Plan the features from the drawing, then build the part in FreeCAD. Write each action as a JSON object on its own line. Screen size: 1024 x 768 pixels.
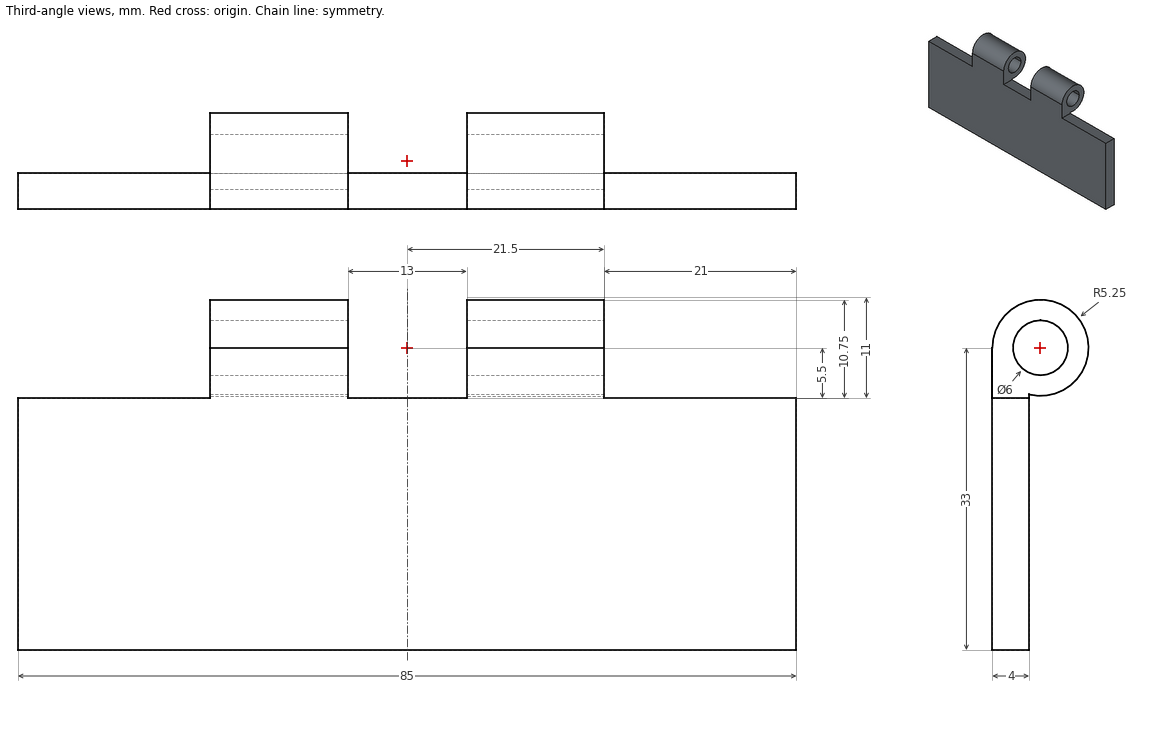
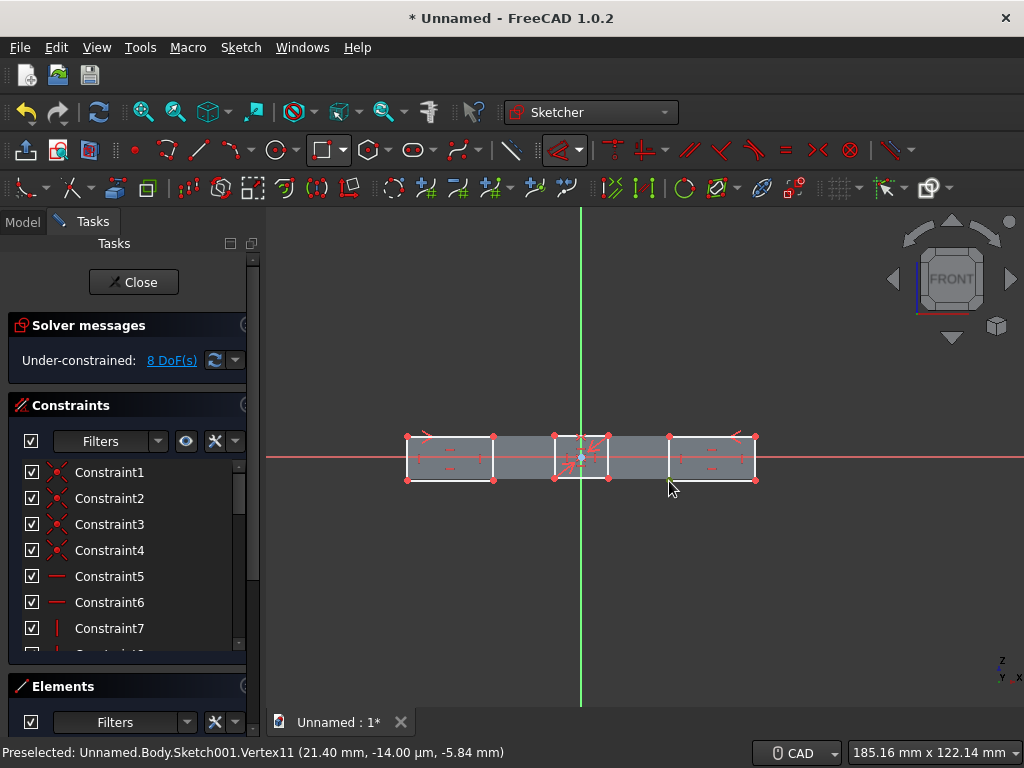
{"action": "left_click", "coordinate": [493, 481]}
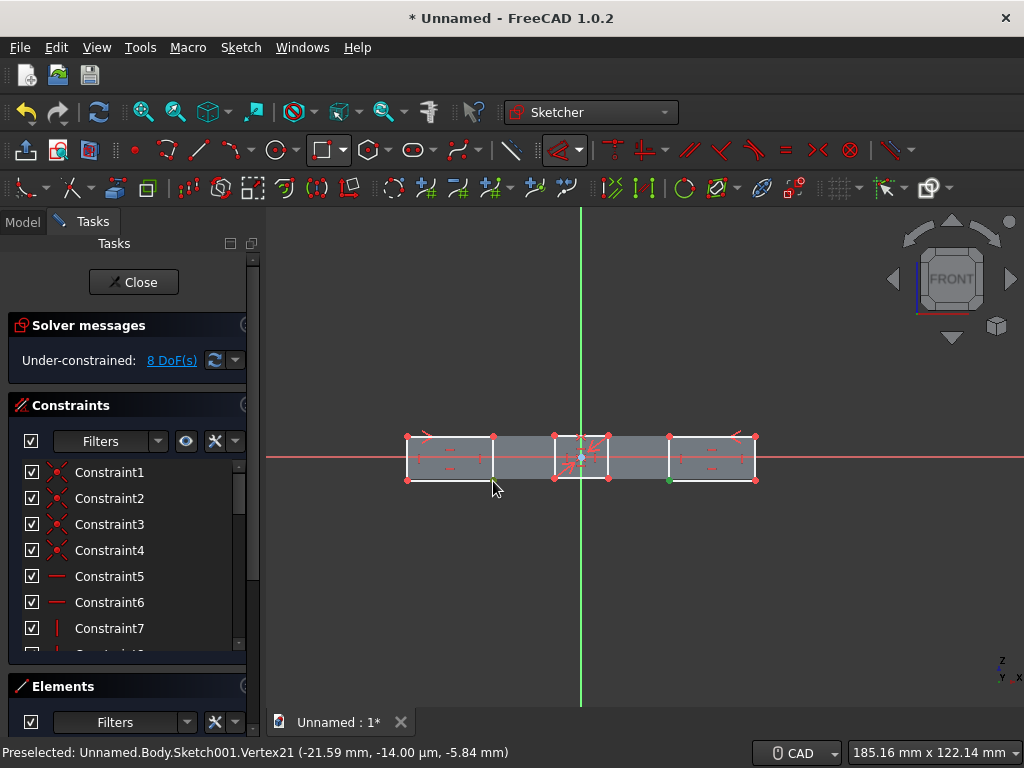
{"action": "left_click", "coordinate": [581, 647]}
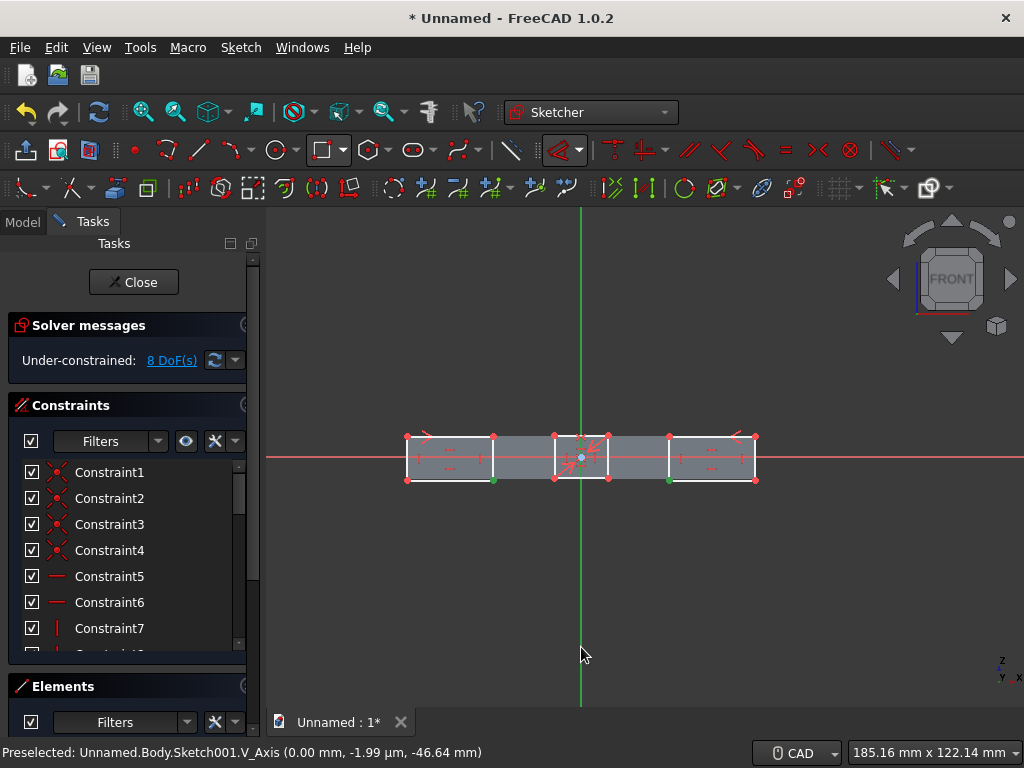
{"action": "left_click", "coordinate": [818, 150]}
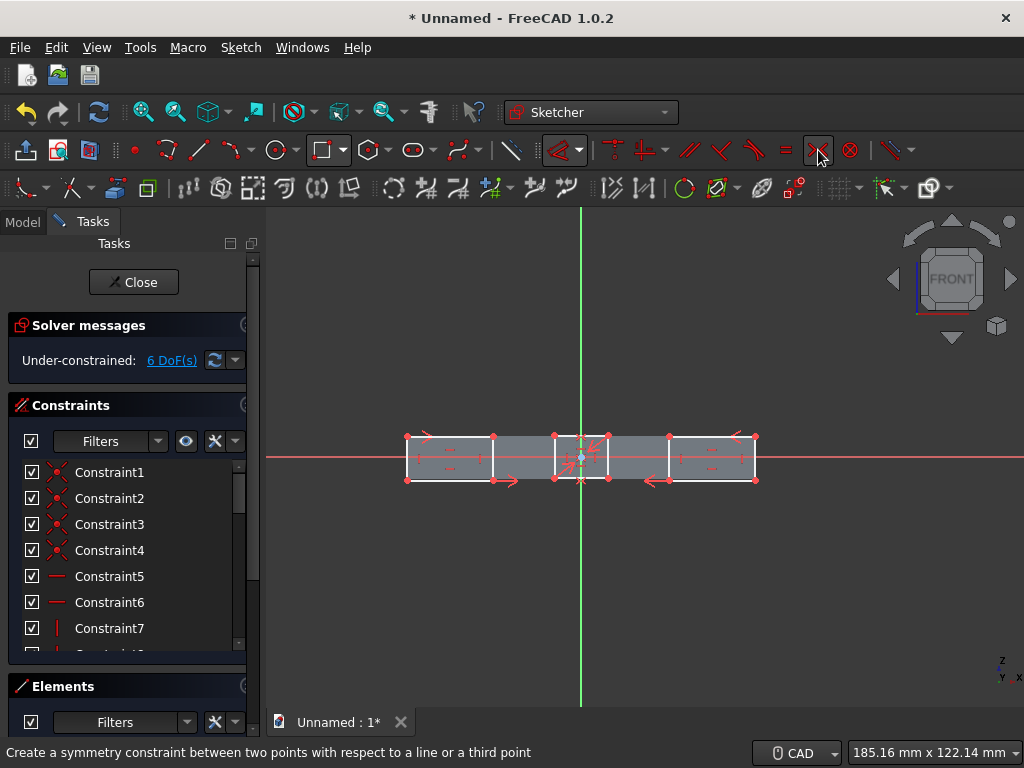
{"action": "scroll", "coordinate": [571, 478], "scroll_direction": "up", "scroll_amount": 2}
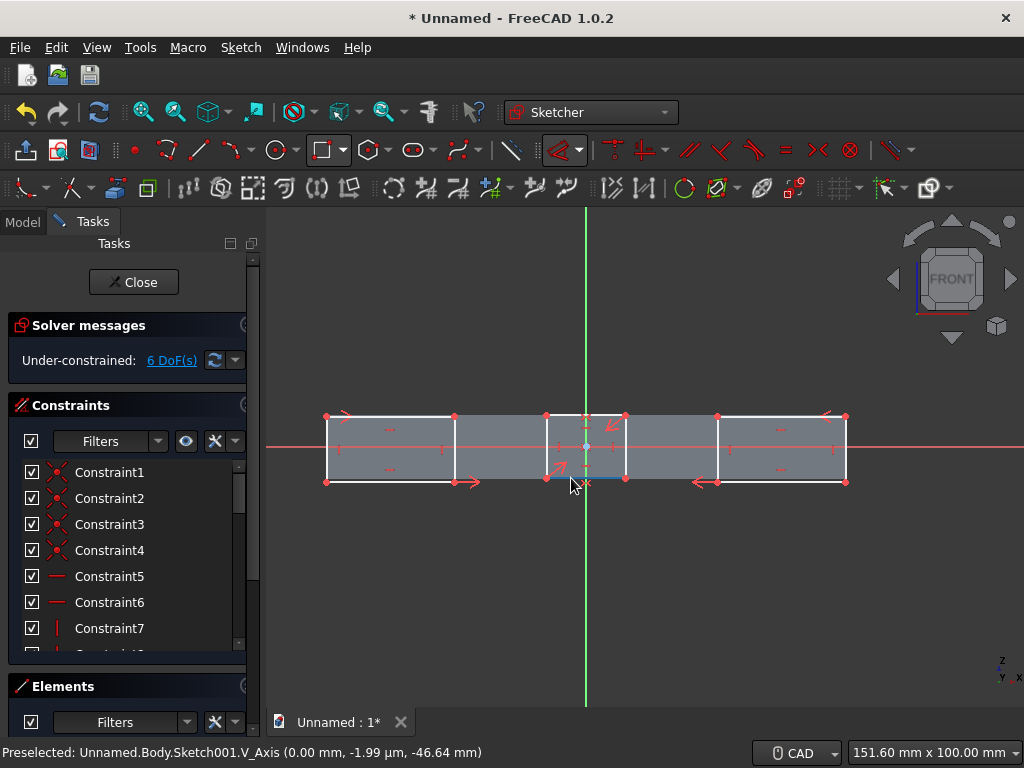
{"action": "left_click", "coordinate": [570, 478]}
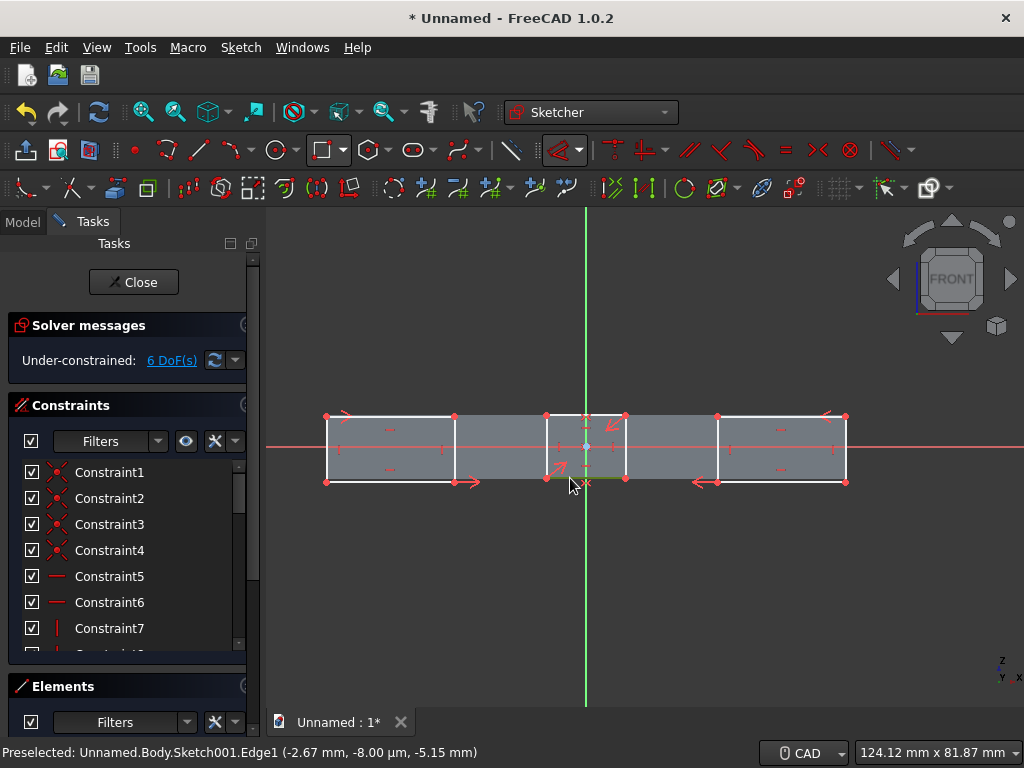
{"action": "key", "text": "l"}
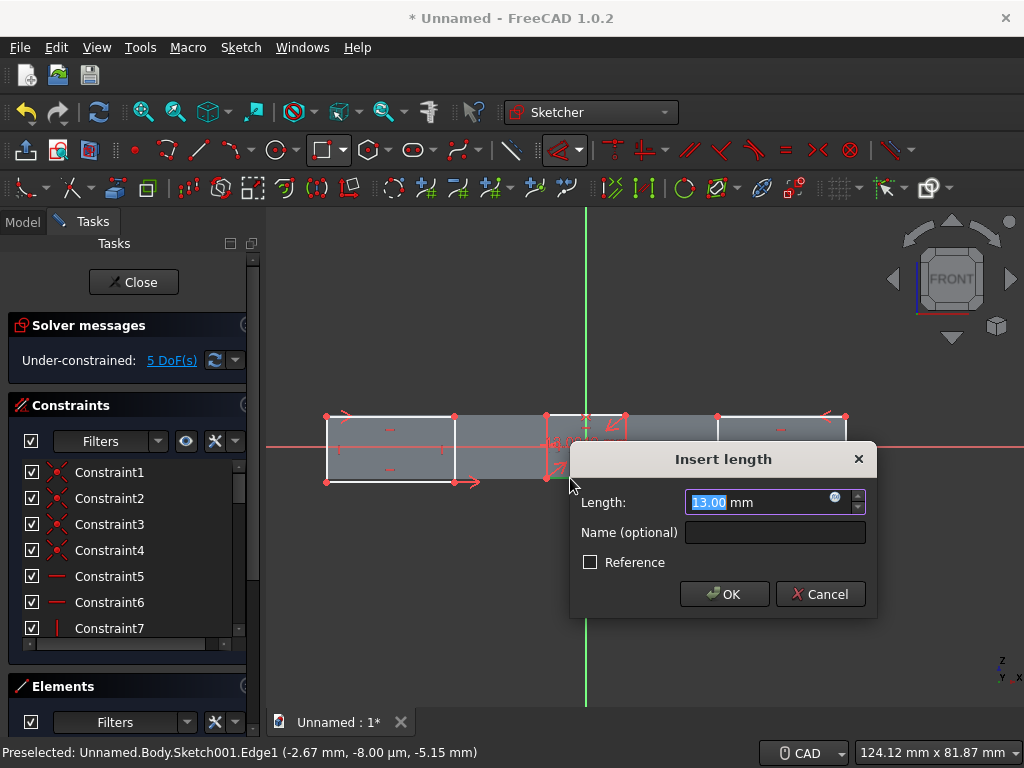
{"action": "type", "text": "13"}
{"action": "key", "text": "Return"}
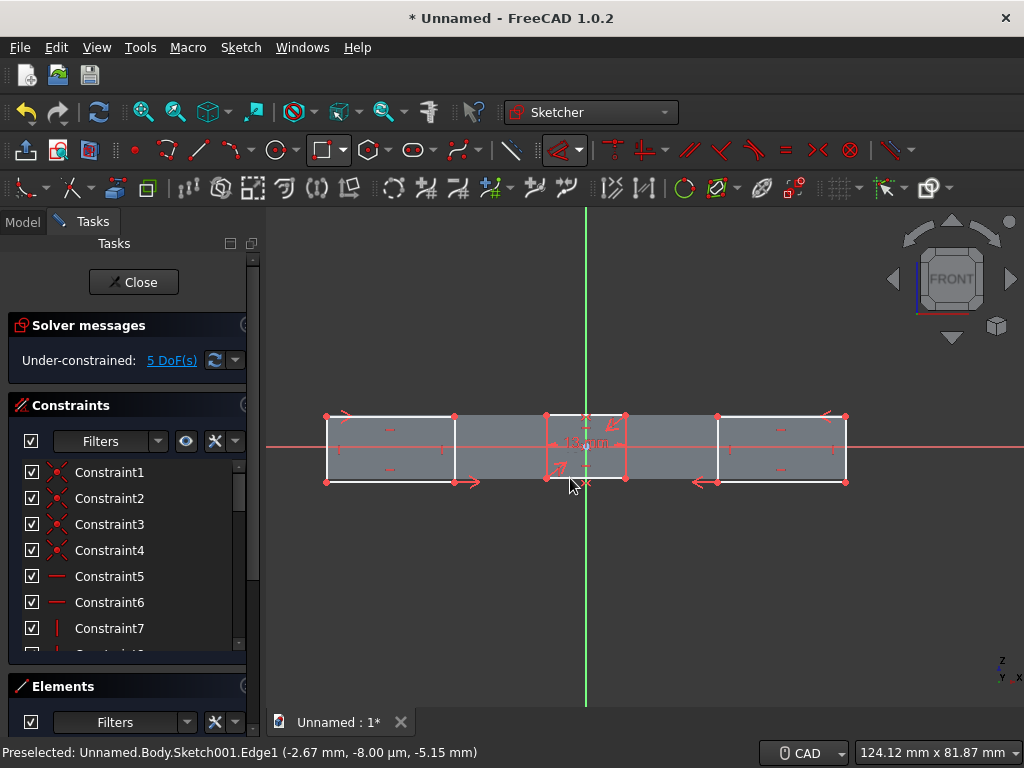
{"action": "left_click", "coordinate": [626, 459]}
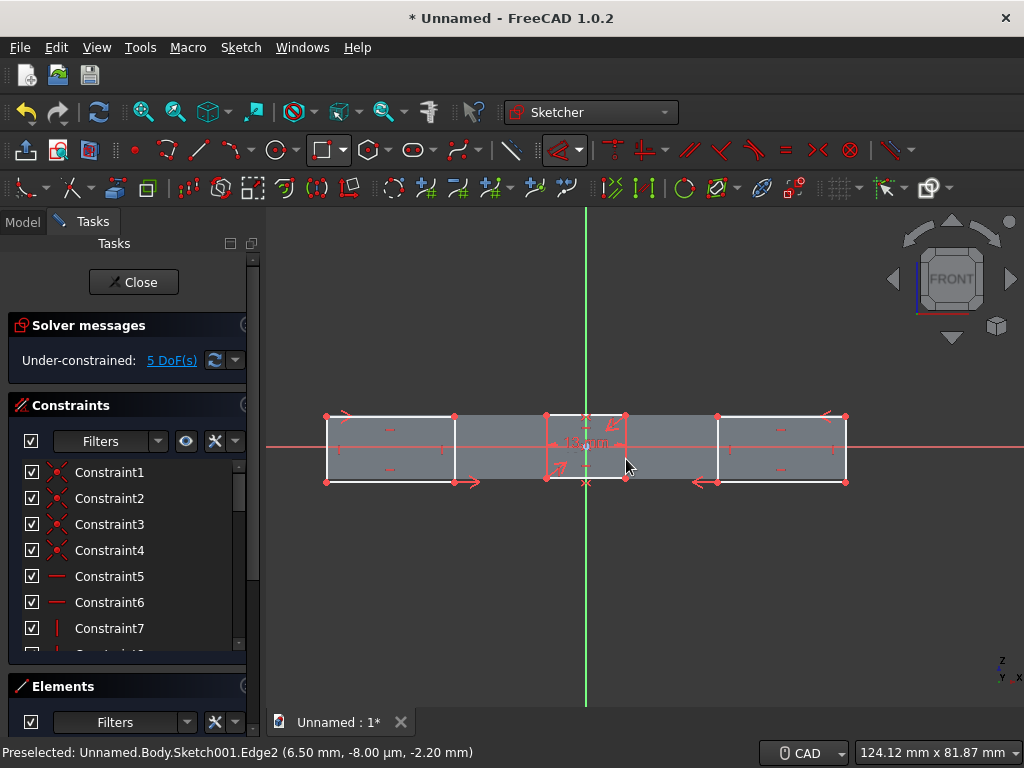
{"action": "left_click", "coordinate": [582, 150]}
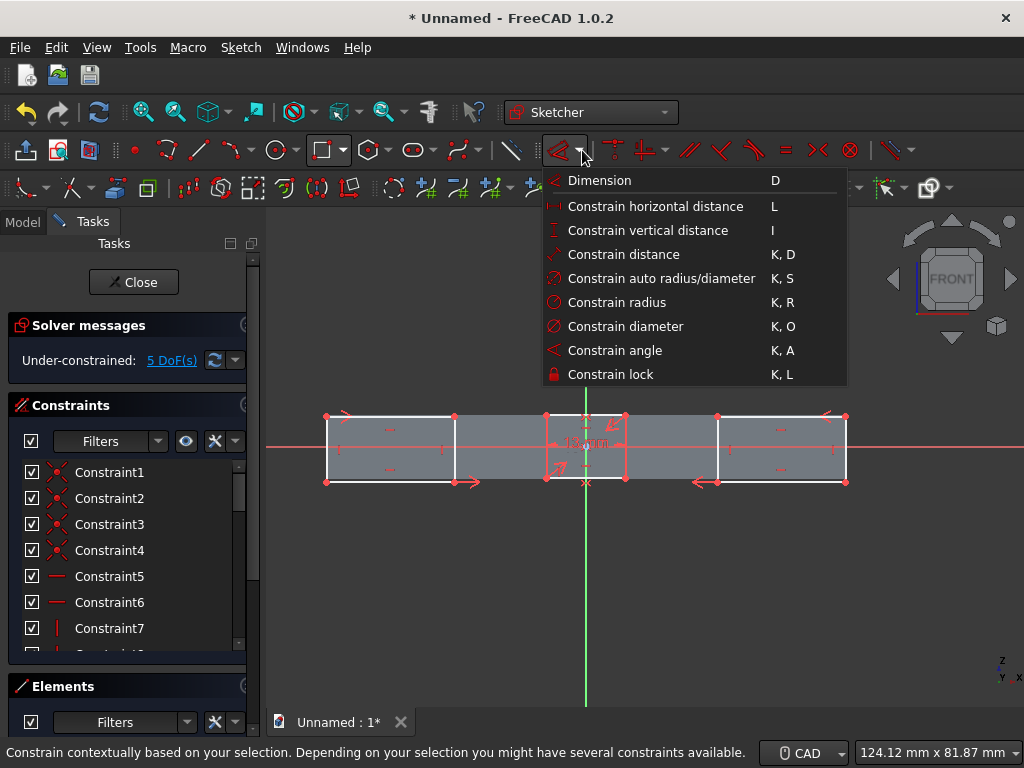
{"action": "left_click", "coordinate": [695, 230]}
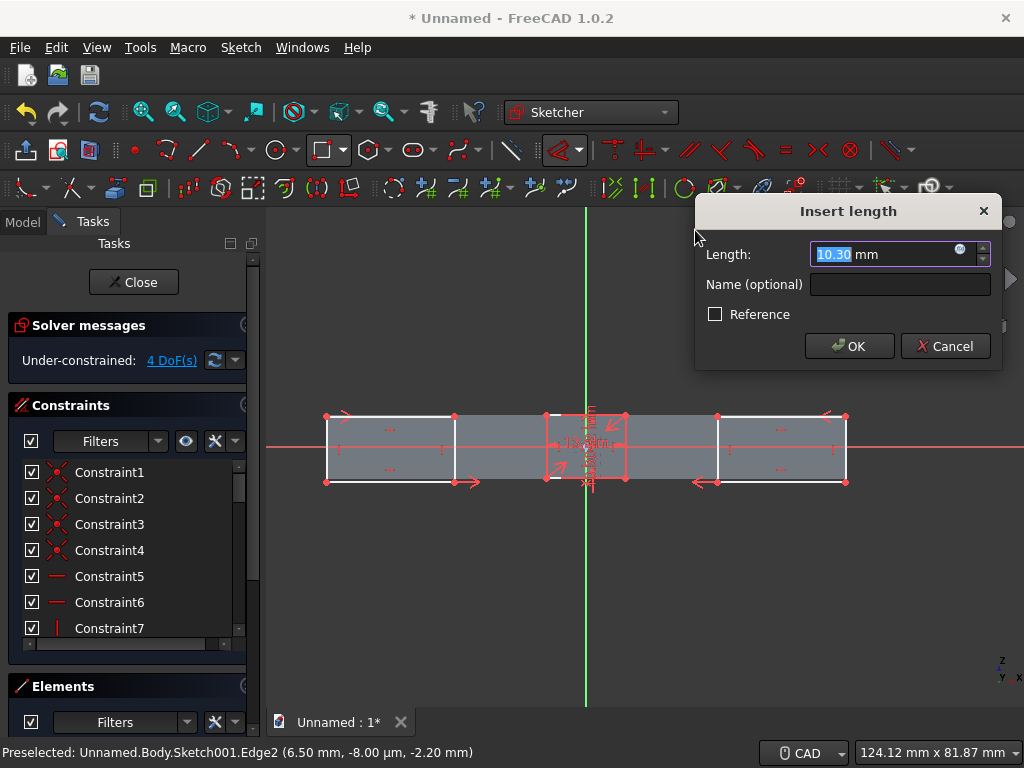
{"action": "type", "text": "11"}
{"action": "key", "text": "Return"}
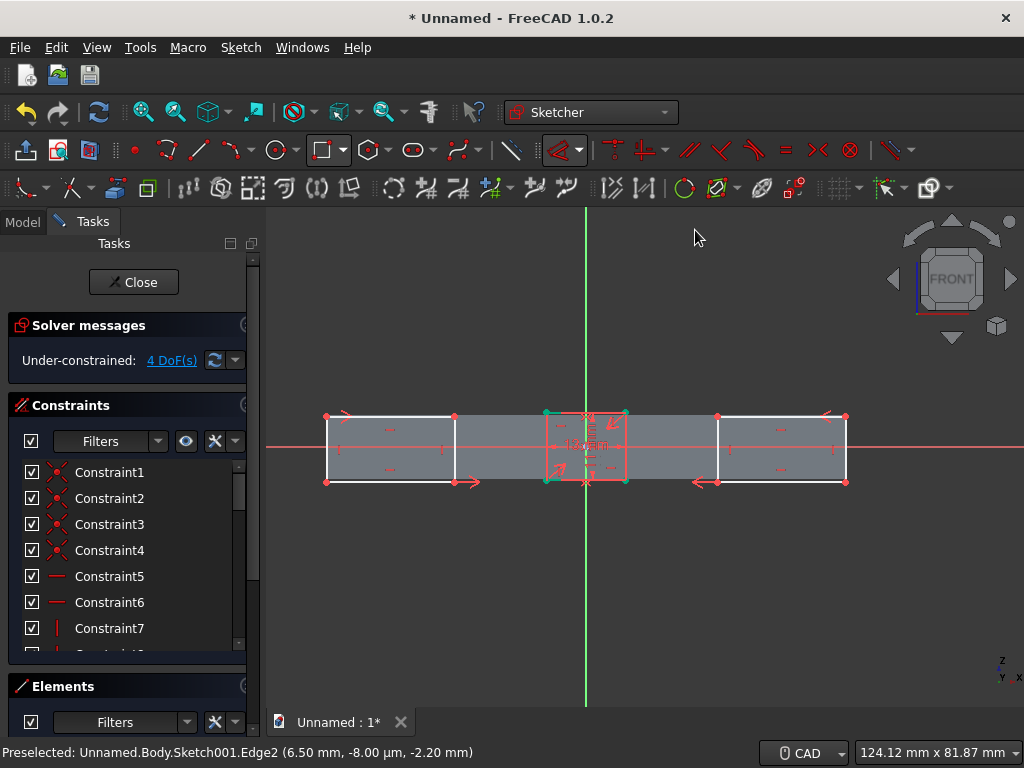
{"action": "left_click", "coordinate": [756, 482]}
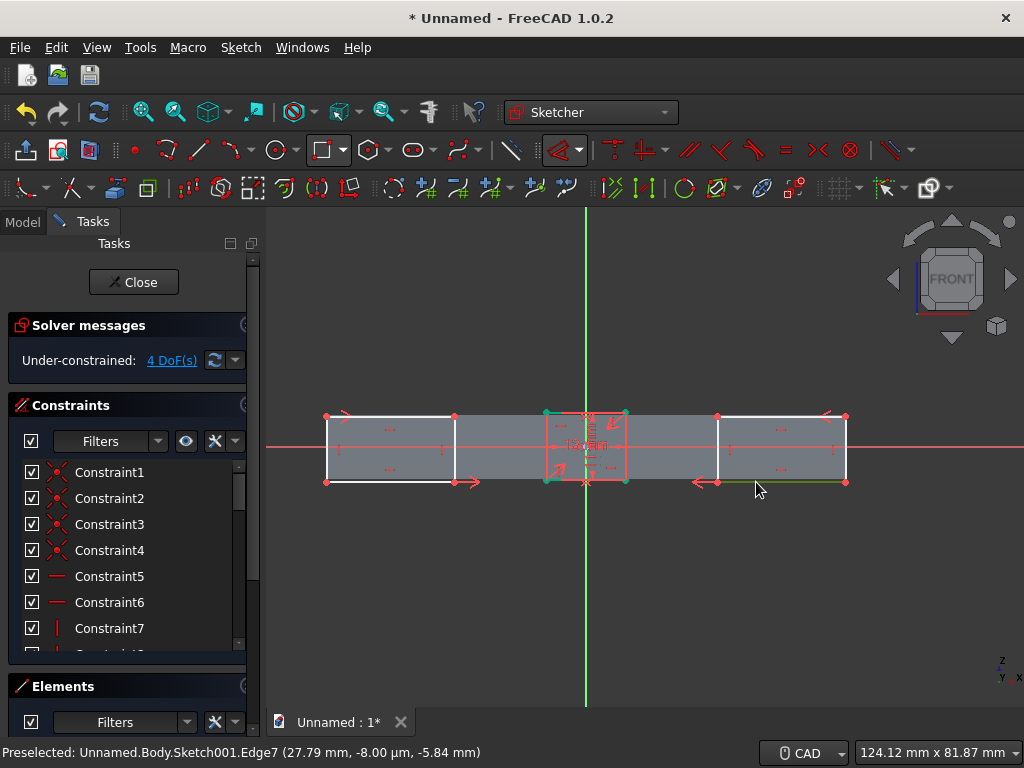
{"action": "key", "text": "l"}